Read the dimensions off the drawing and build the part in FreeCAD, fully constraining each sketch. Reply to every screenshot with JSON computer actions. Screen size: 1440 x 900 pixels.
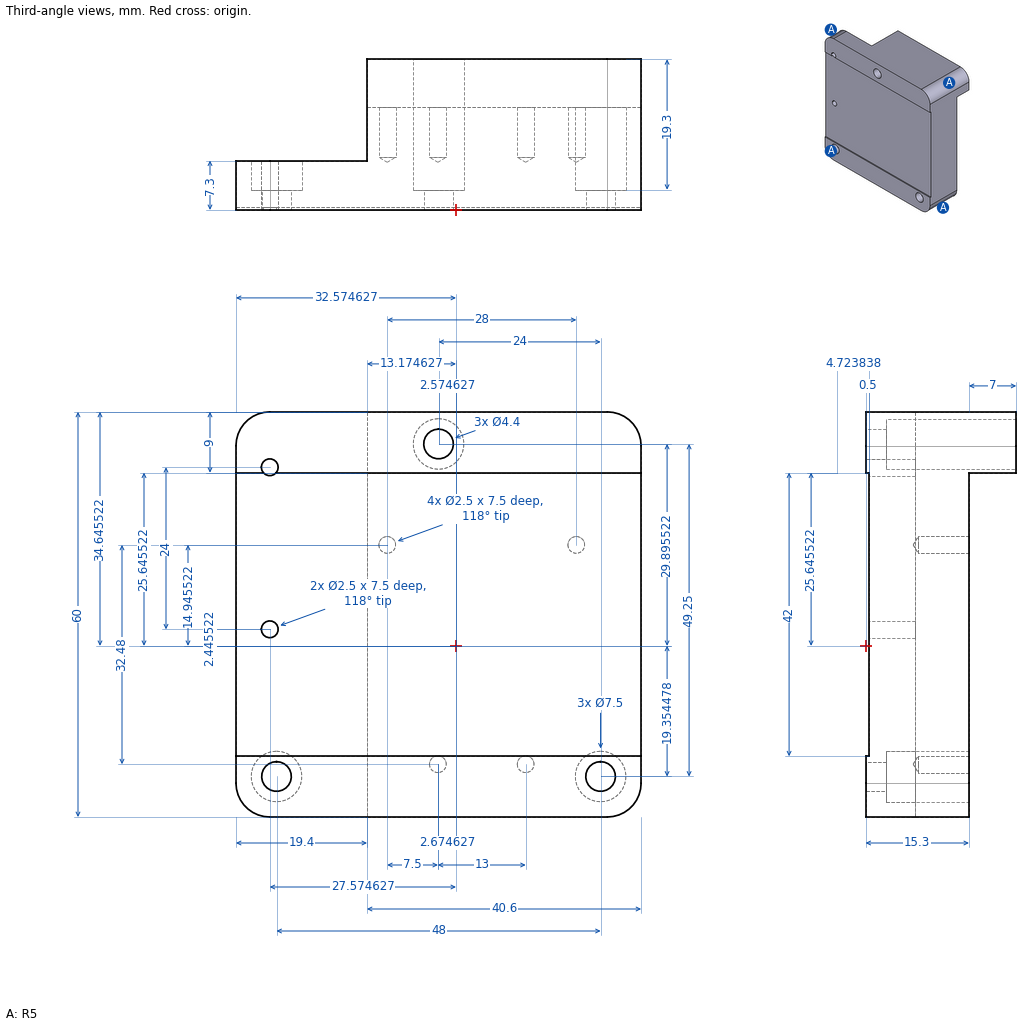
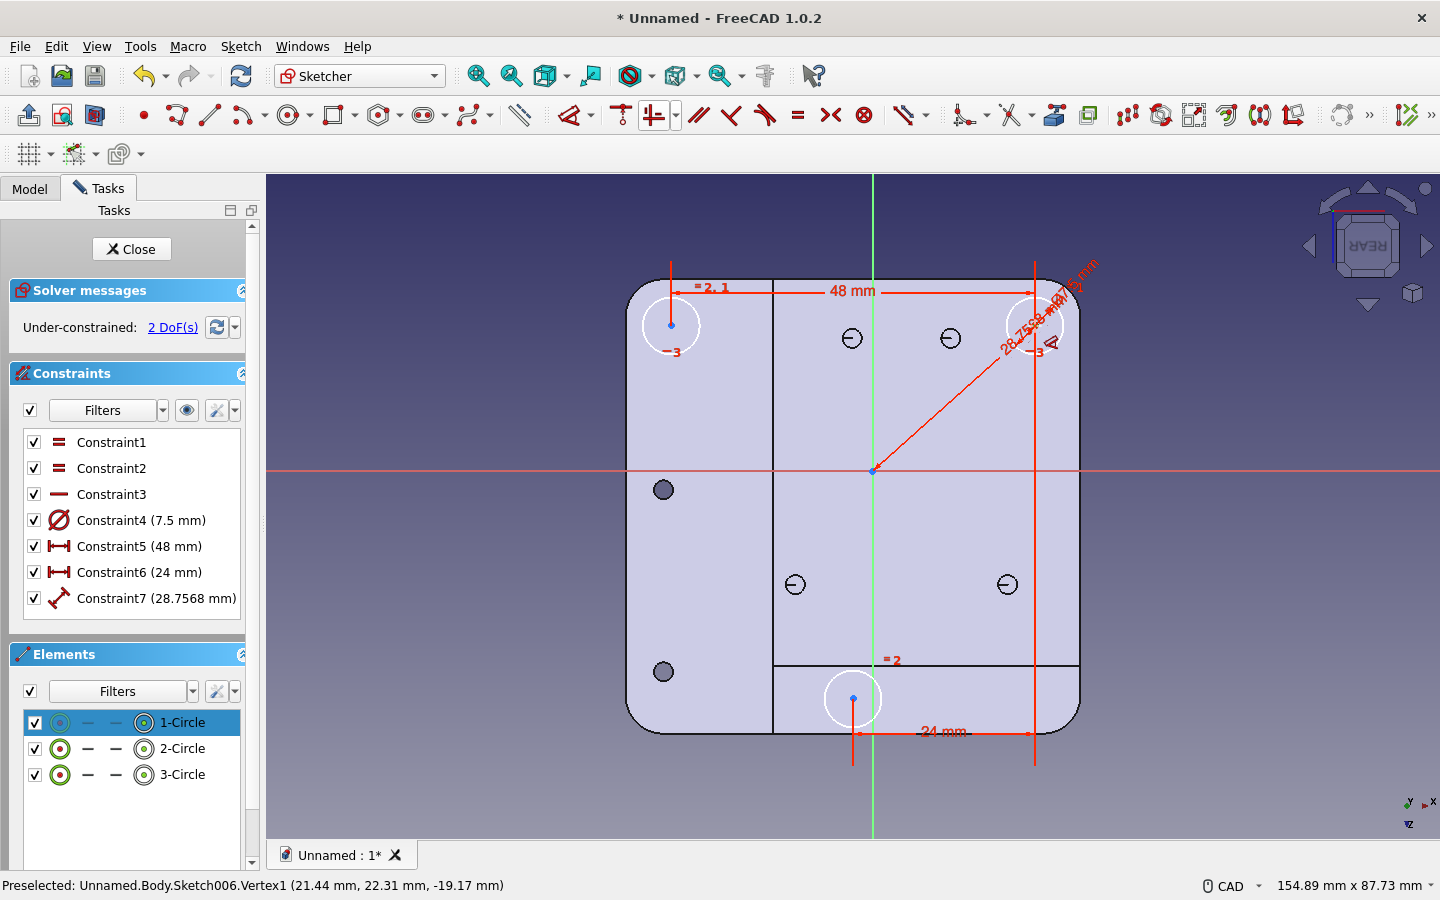
{"action": "left_click", "coordinate": [853, 699]}
{"action": "left_click", "coordinate": [1069, 512]}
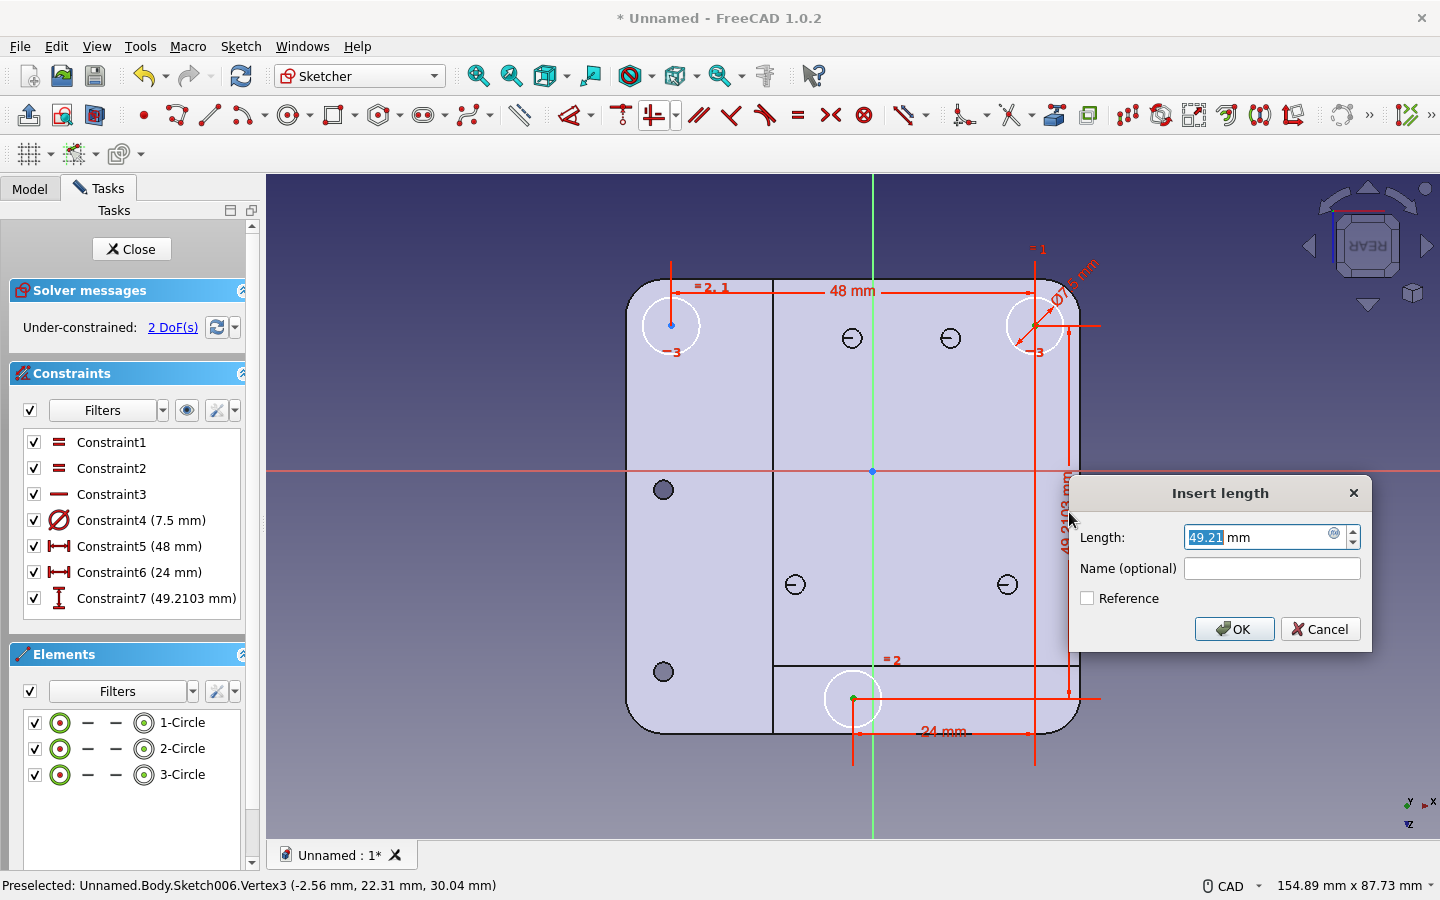
{"action": "type", "text": "49.25"}
{"action": "key", "text": "Return"}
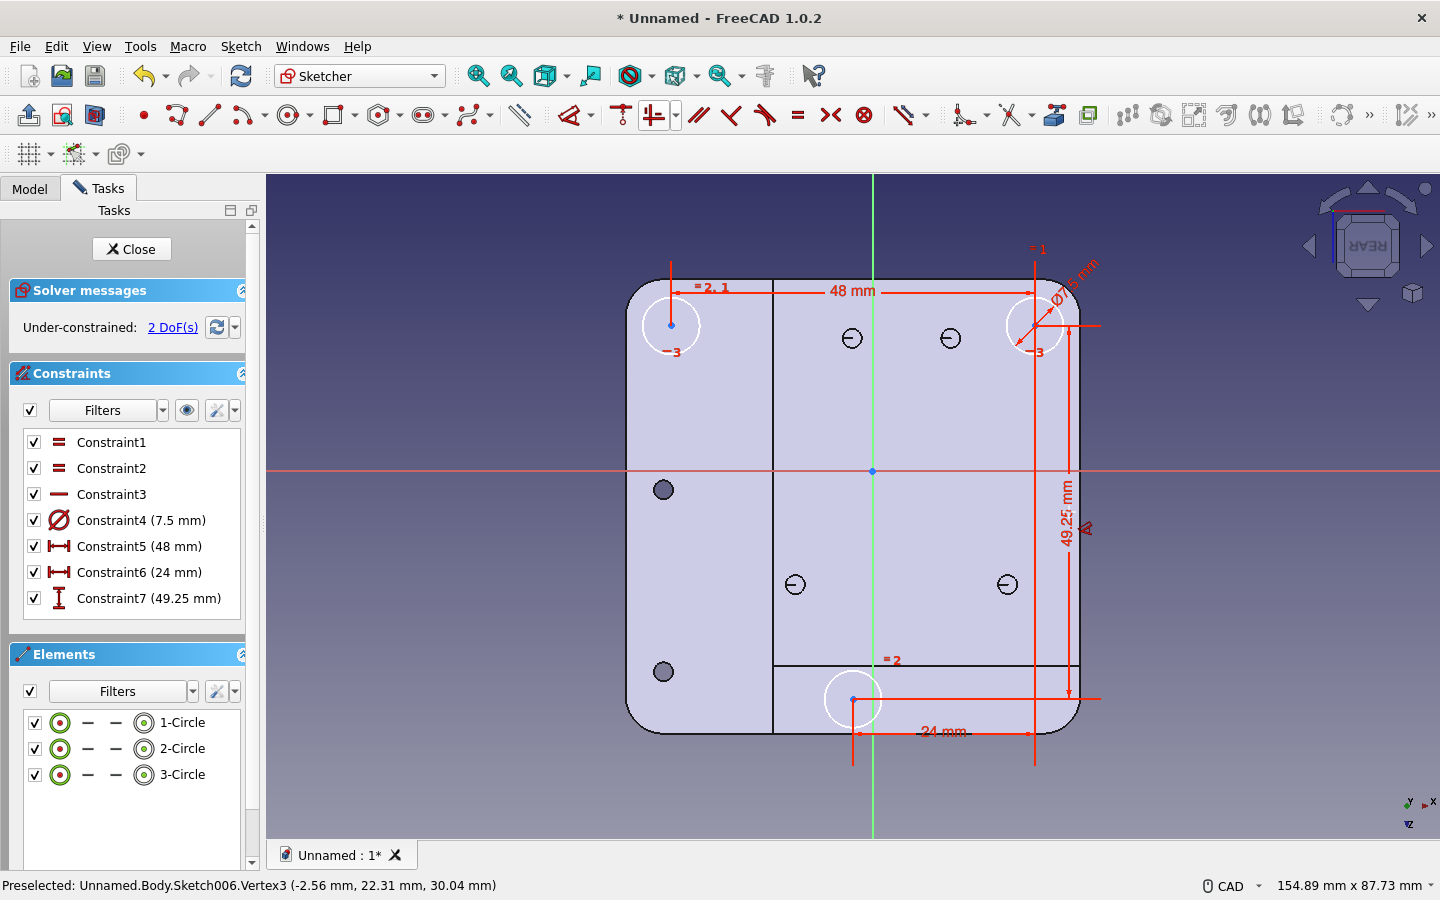
{"action": "scroll", "coordinate": [853, 699], "scroll_direction": "up", "scroll_amount": 4}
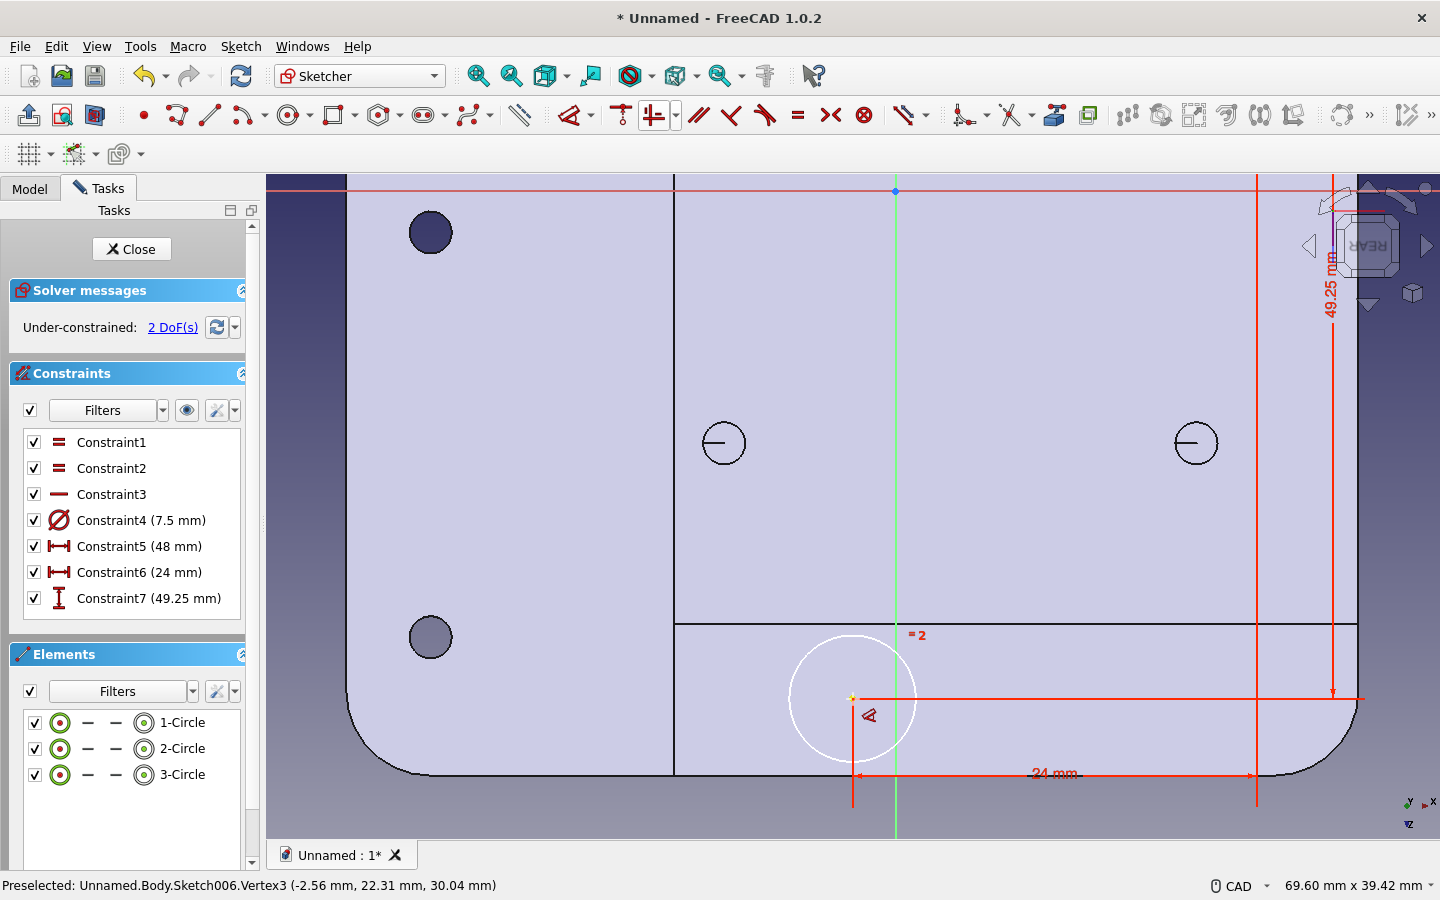
{"action": "left_click", "coordinate": [853, 699]}
{"action": "left_click", "coordinate": [874, 733]}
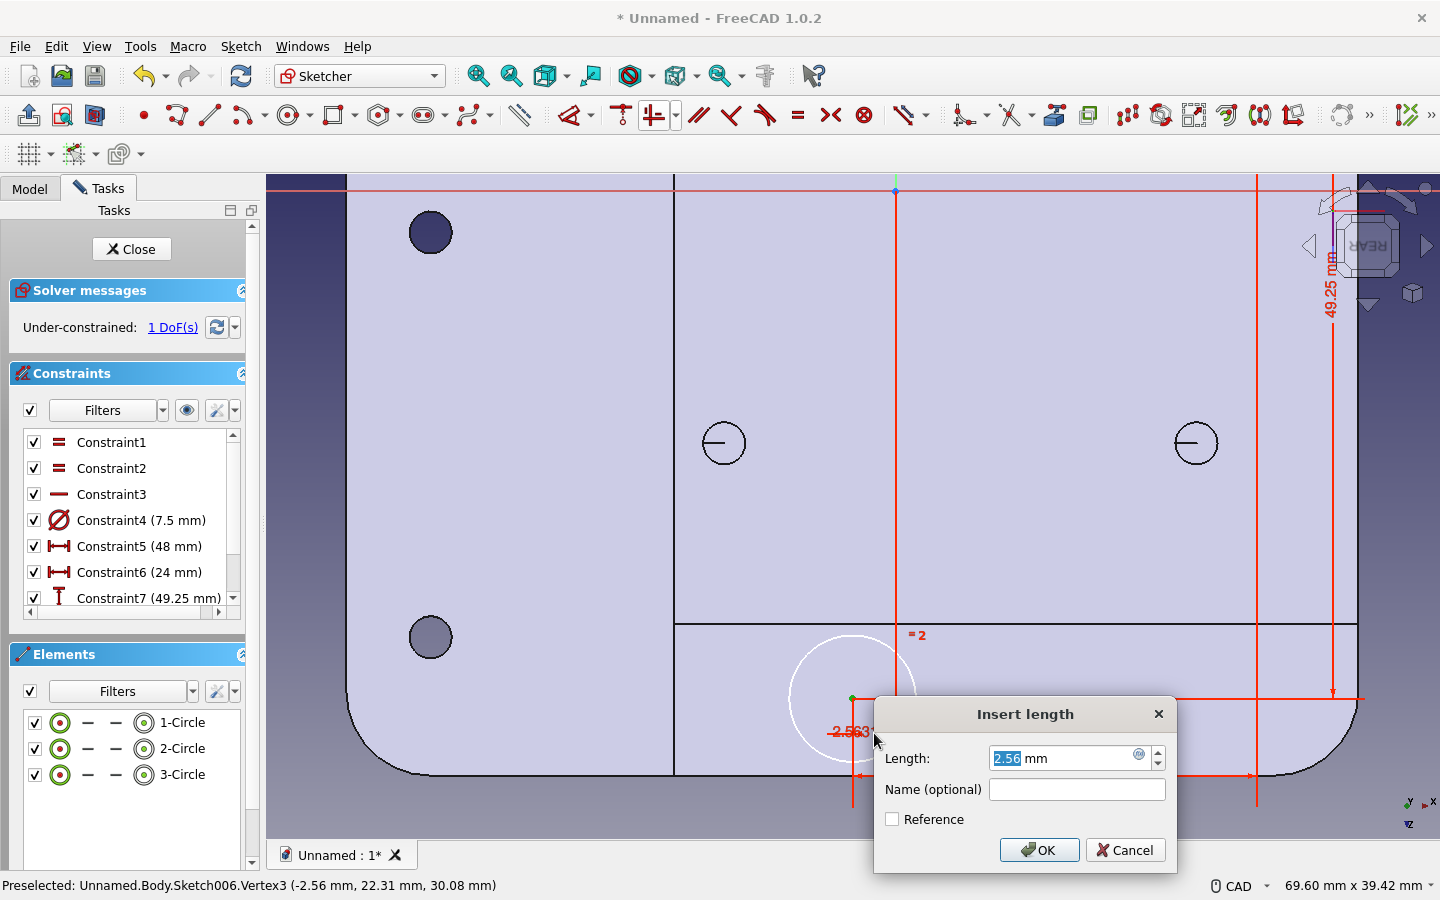
{"action": "type", "text": "2.574627"}
{"action": "key", "text": "Return"}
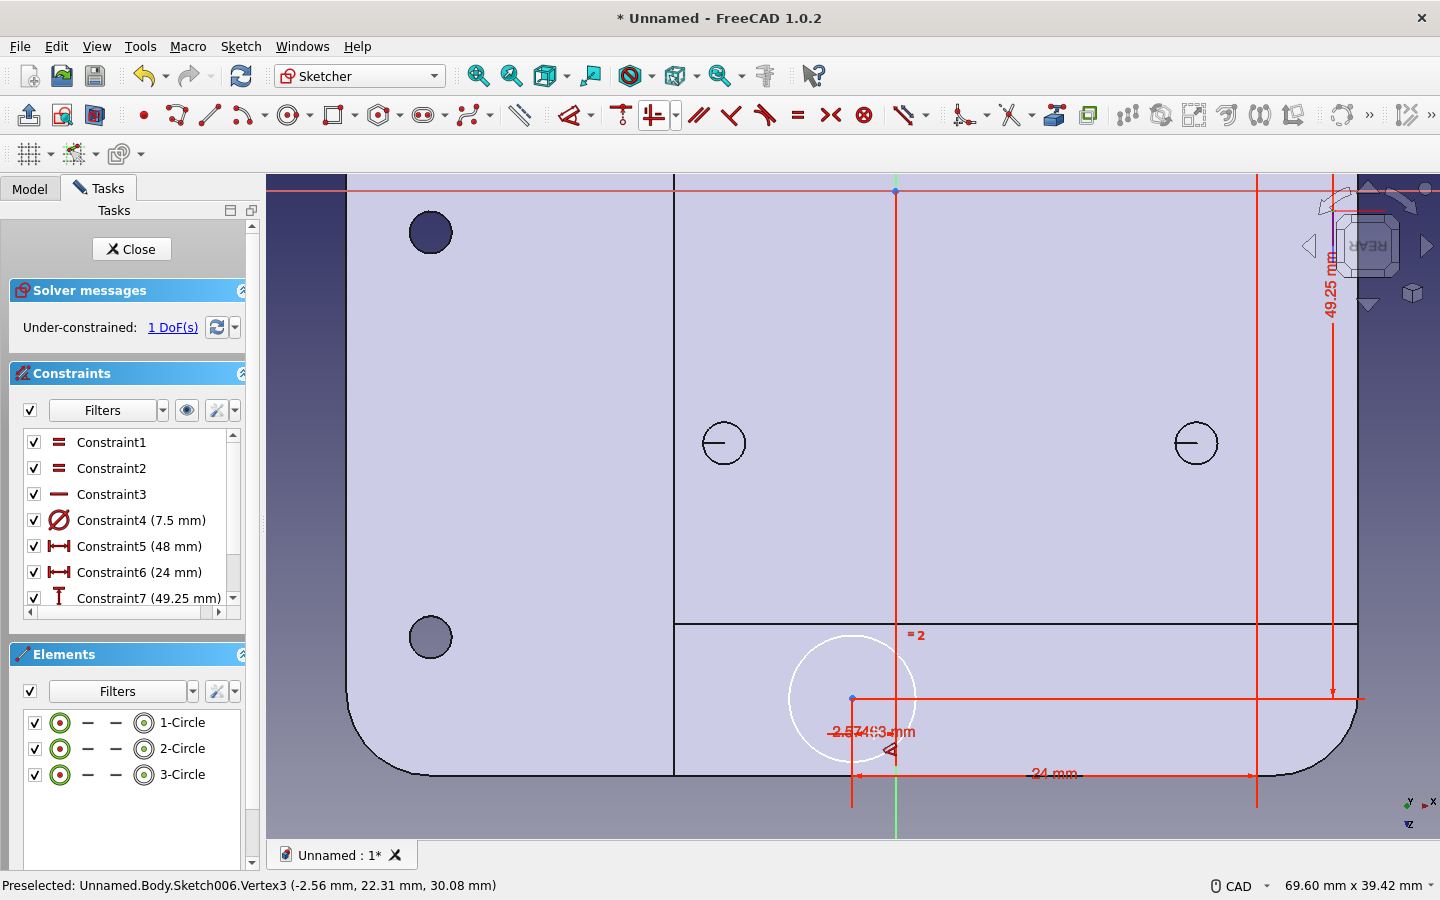
{"action": "scroll", "coordinate": [729, 691], "scroll_direction": "down", "scroll_amount": 4}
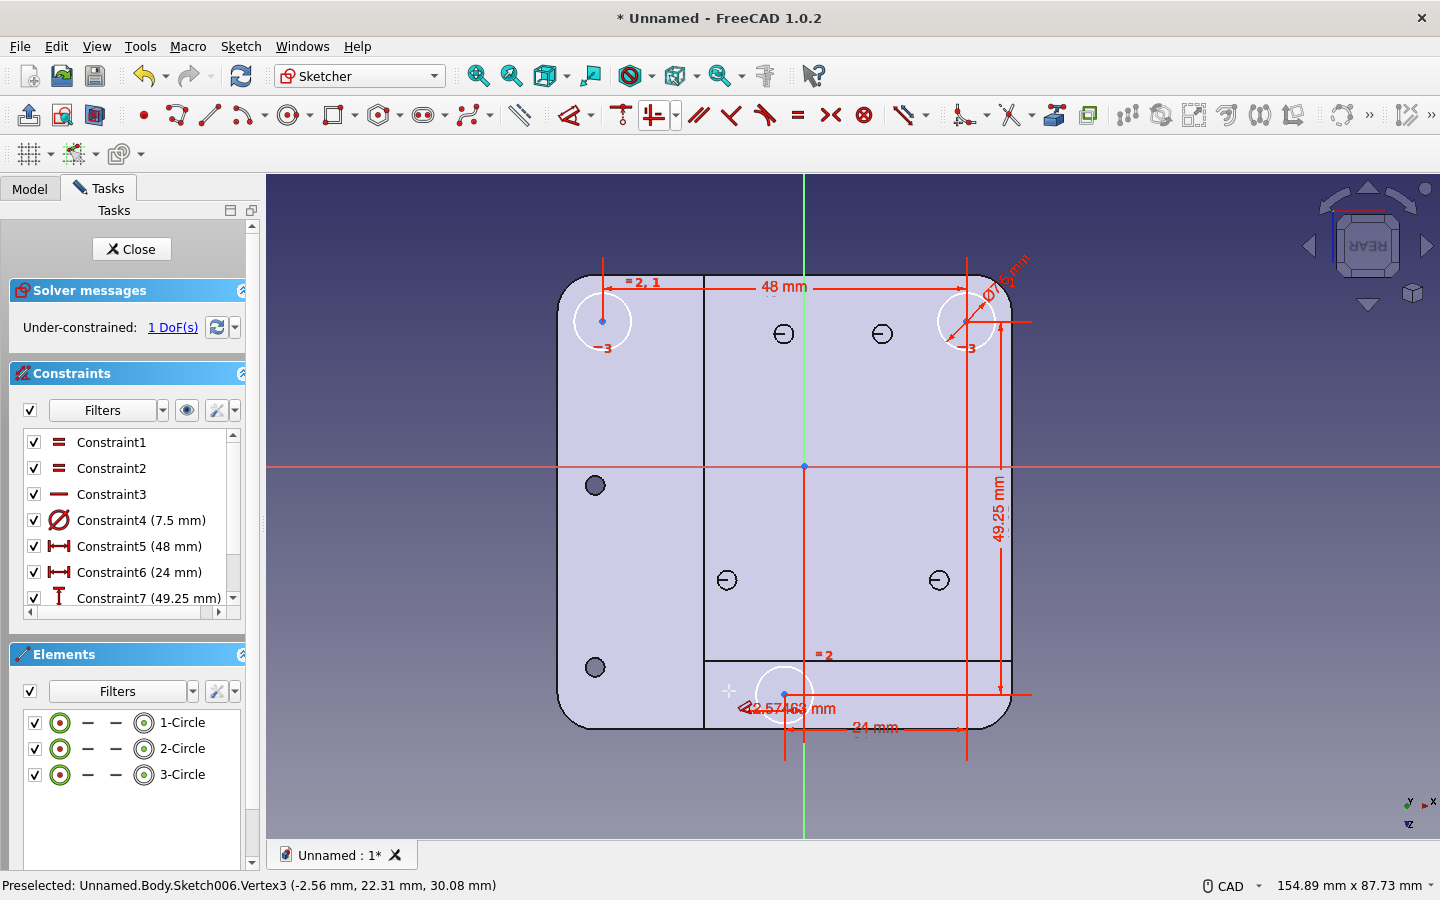
{"action": "left_click", "coordinate": [967, 322]}
{"action": "left_click", "coordinate": [1001, 394]}